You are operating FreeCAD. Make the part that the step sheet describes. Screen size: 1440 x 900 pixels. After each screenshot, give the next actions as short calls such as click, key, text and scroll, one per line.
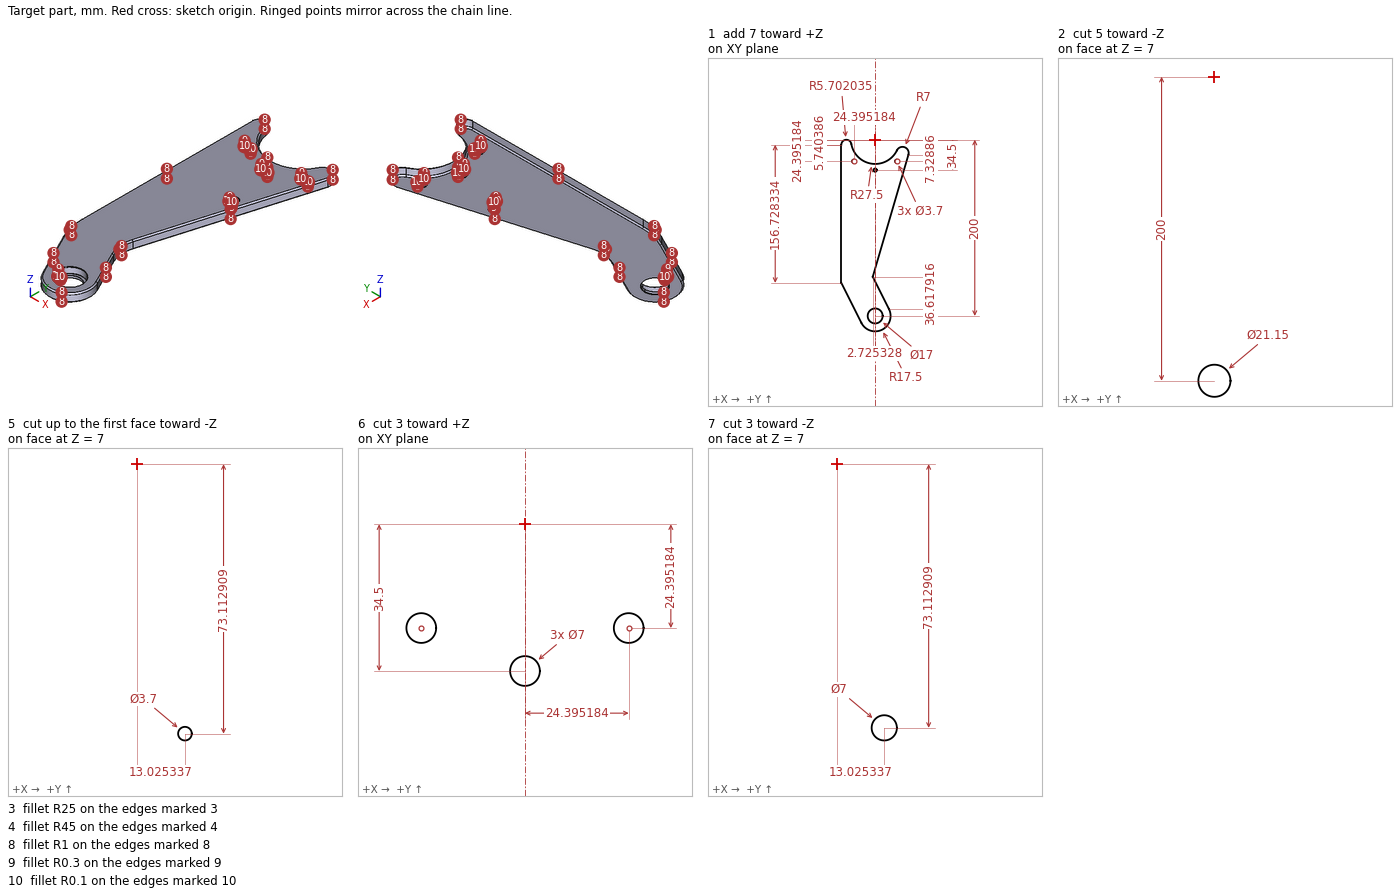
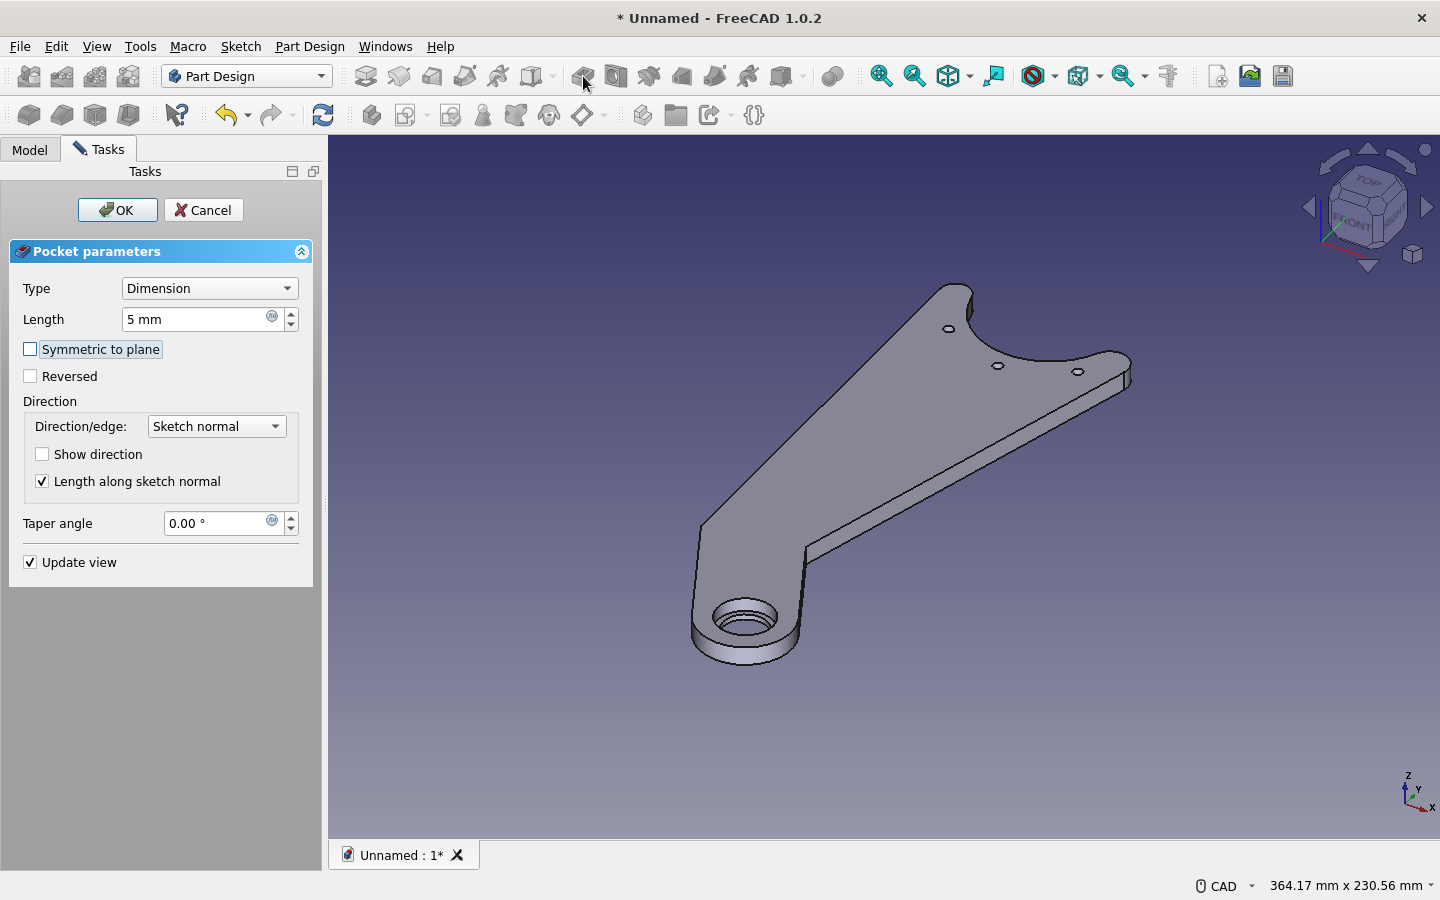
click(118, 210)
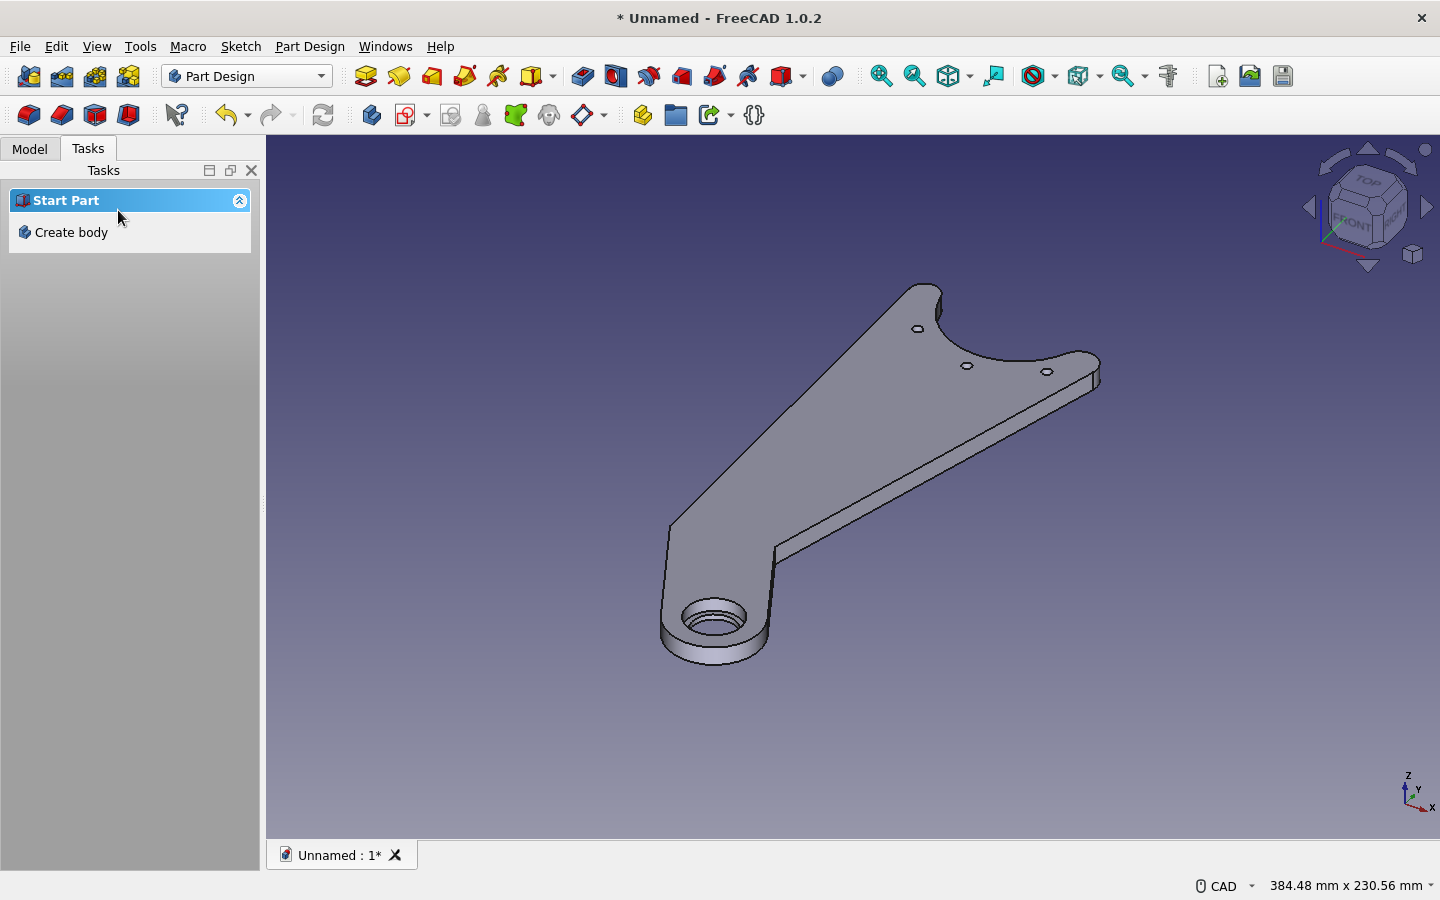
scroll(775, 555, up, 4)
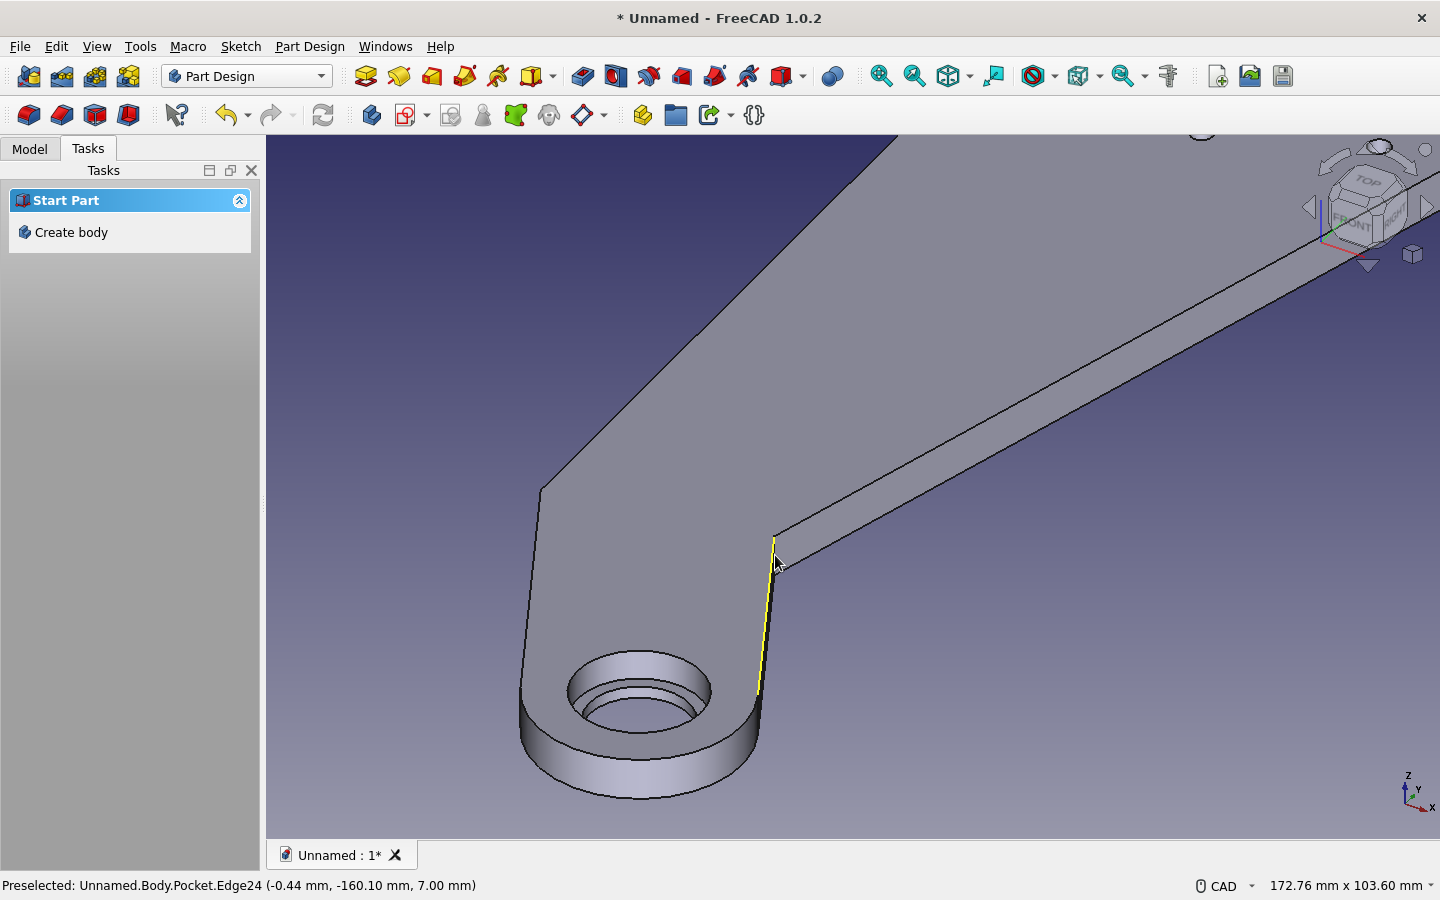
key(v)
key(f)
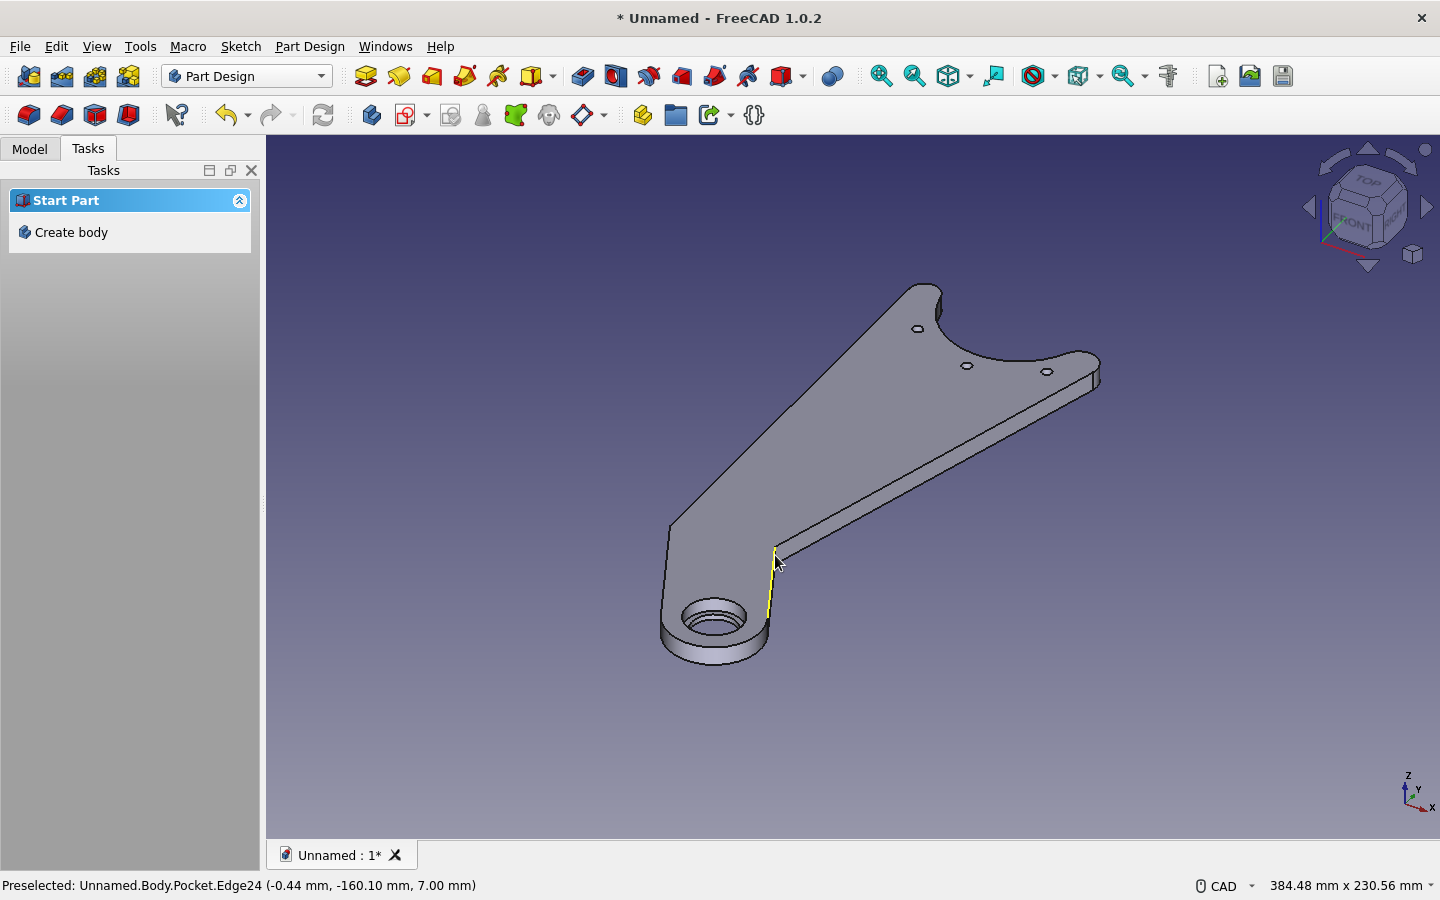
key(0)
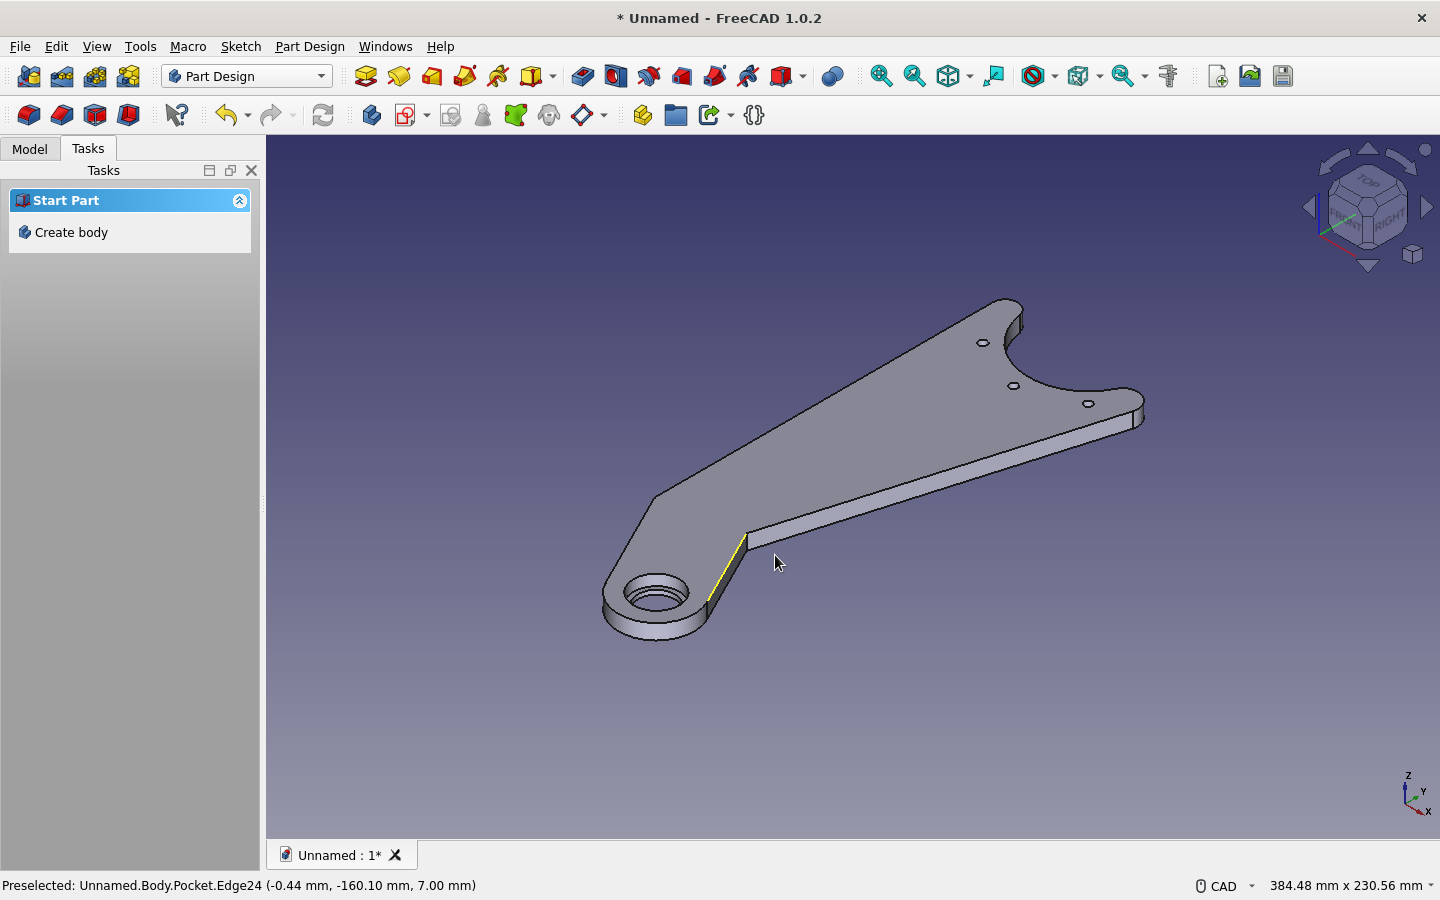
scroll(747, 541, up, 4)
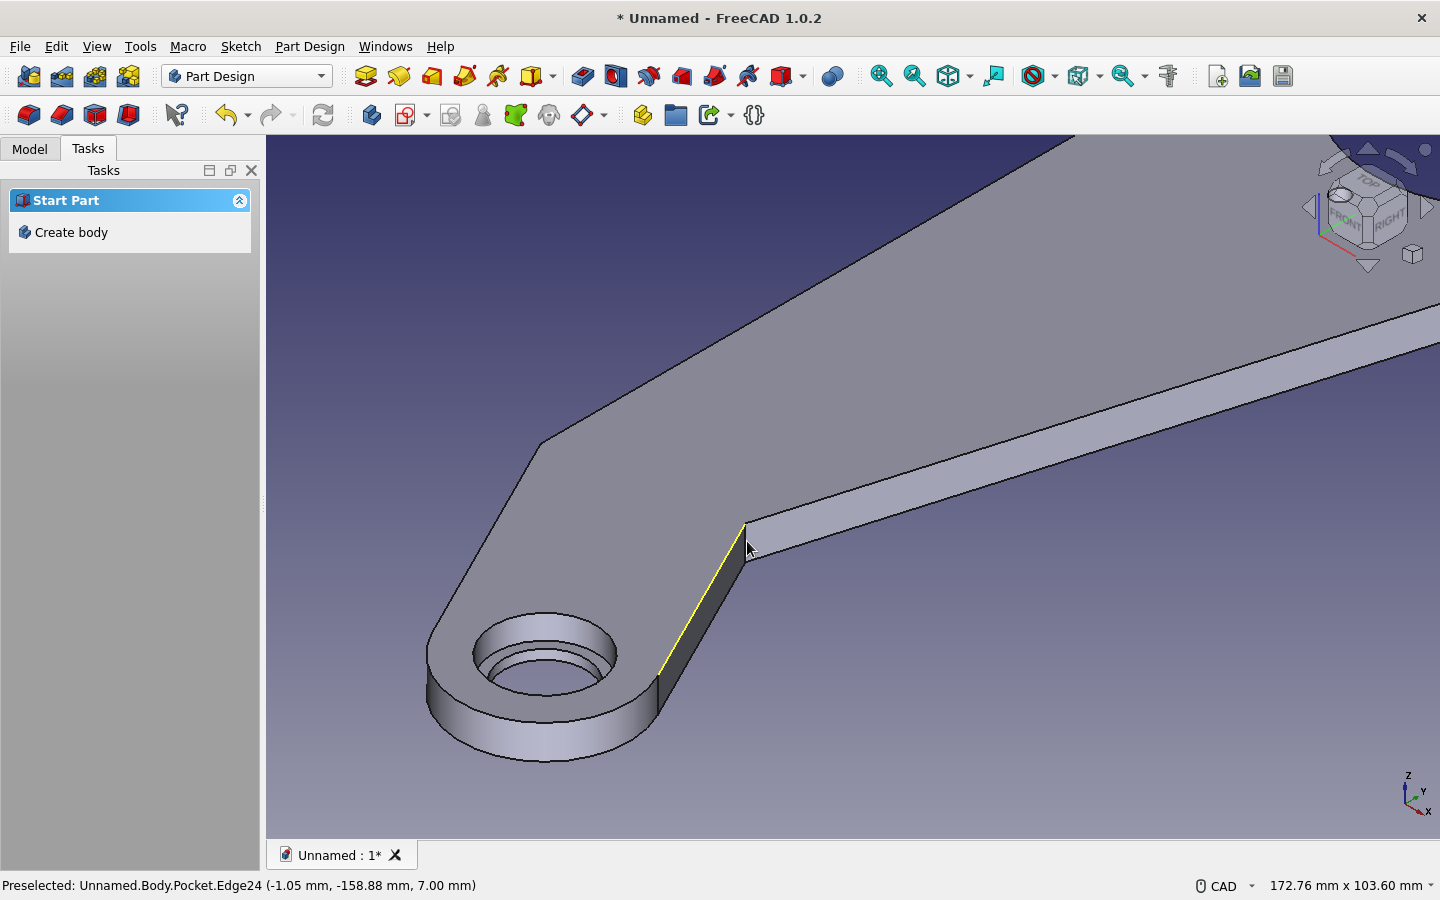
key(v)
key(f)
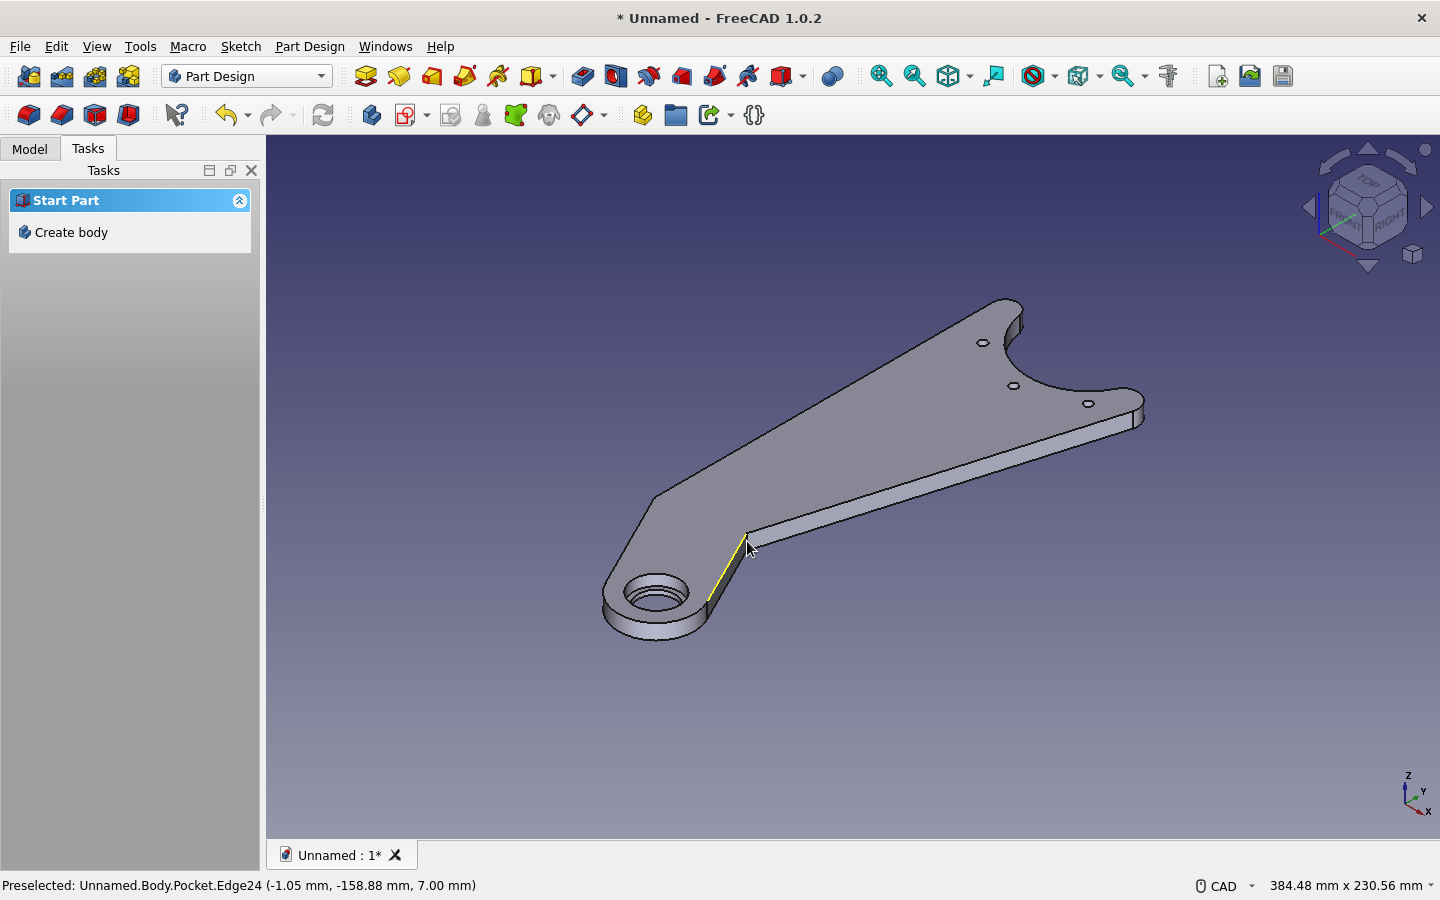
key(2)